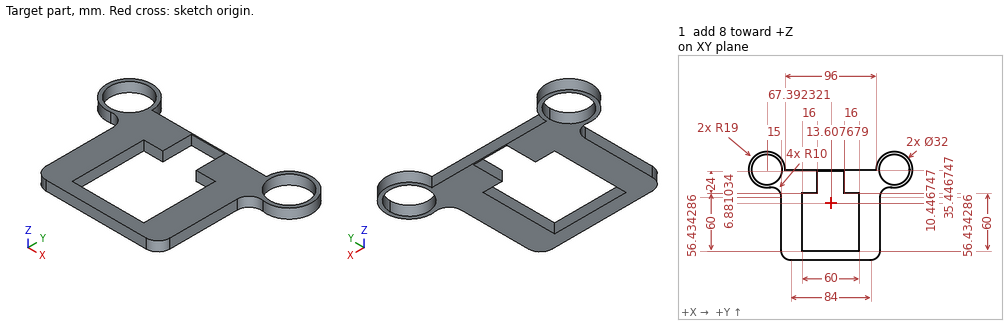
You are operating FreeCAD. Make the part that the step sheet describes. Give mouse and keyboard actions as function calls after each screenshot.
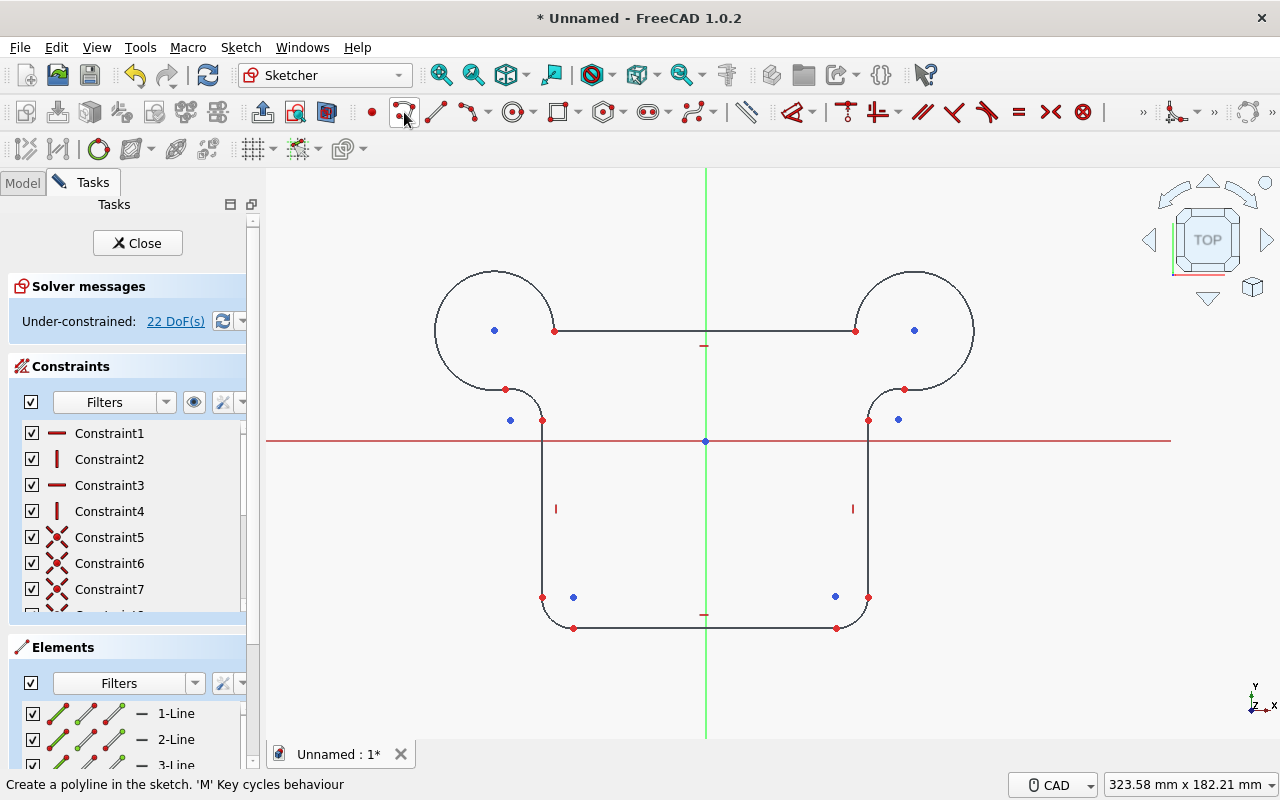
click(749, 409)
click(799, 409)
click(799, 597)
click(611, 597)
click(611, 409)
click(661, 409)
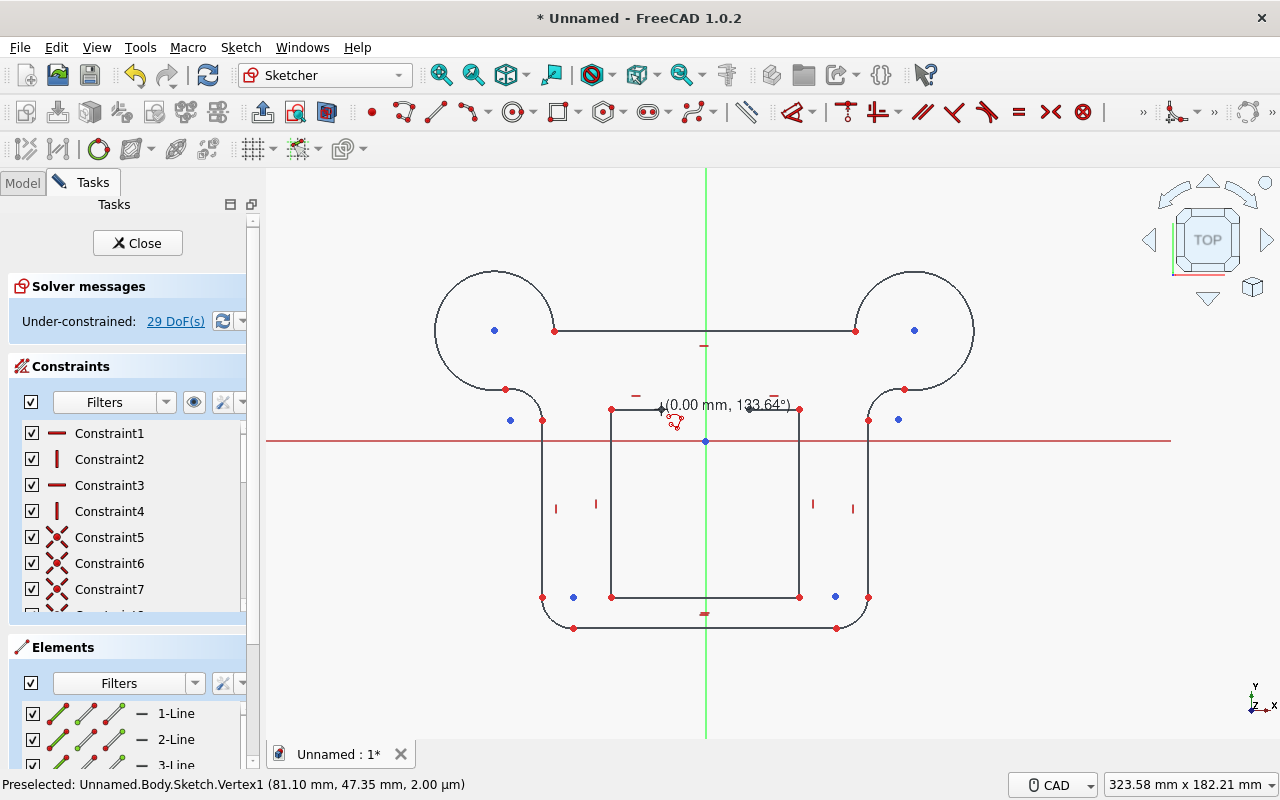
scroll(661, 333, up, 9)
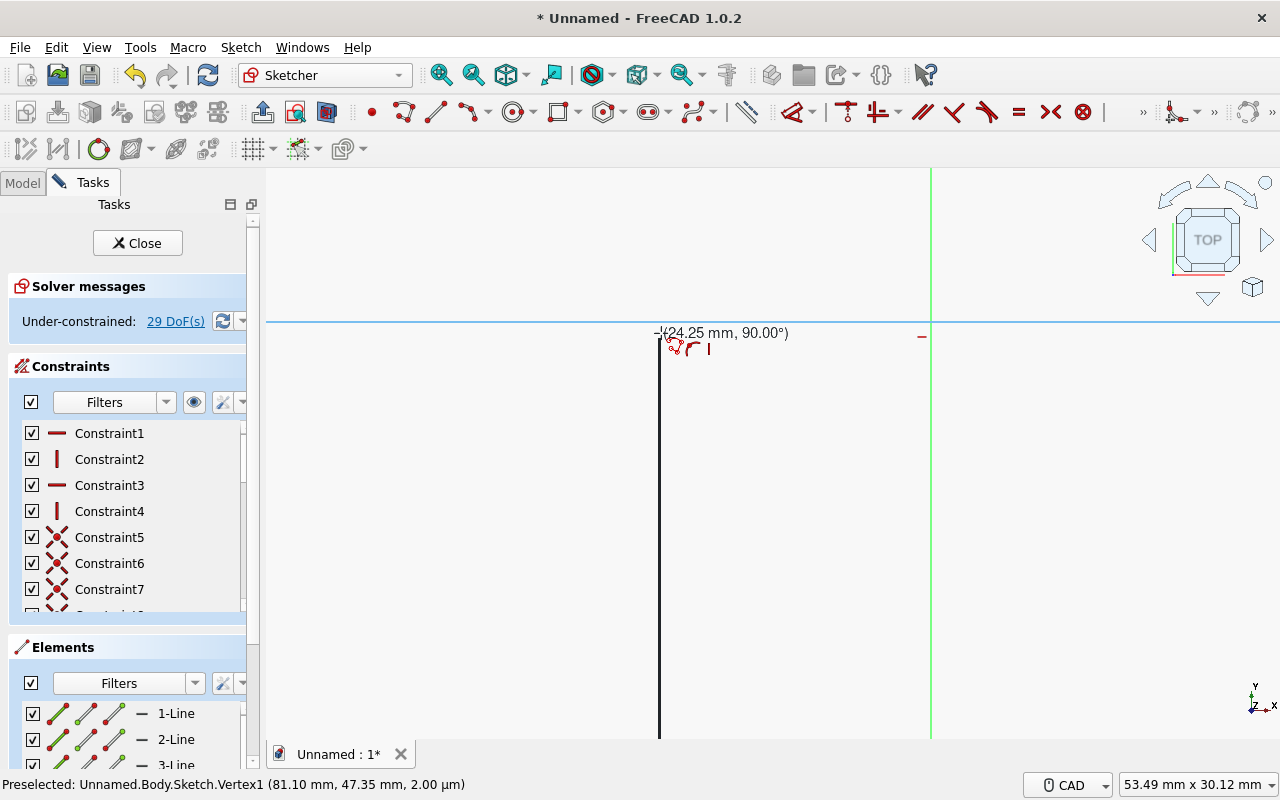
click(659, 334)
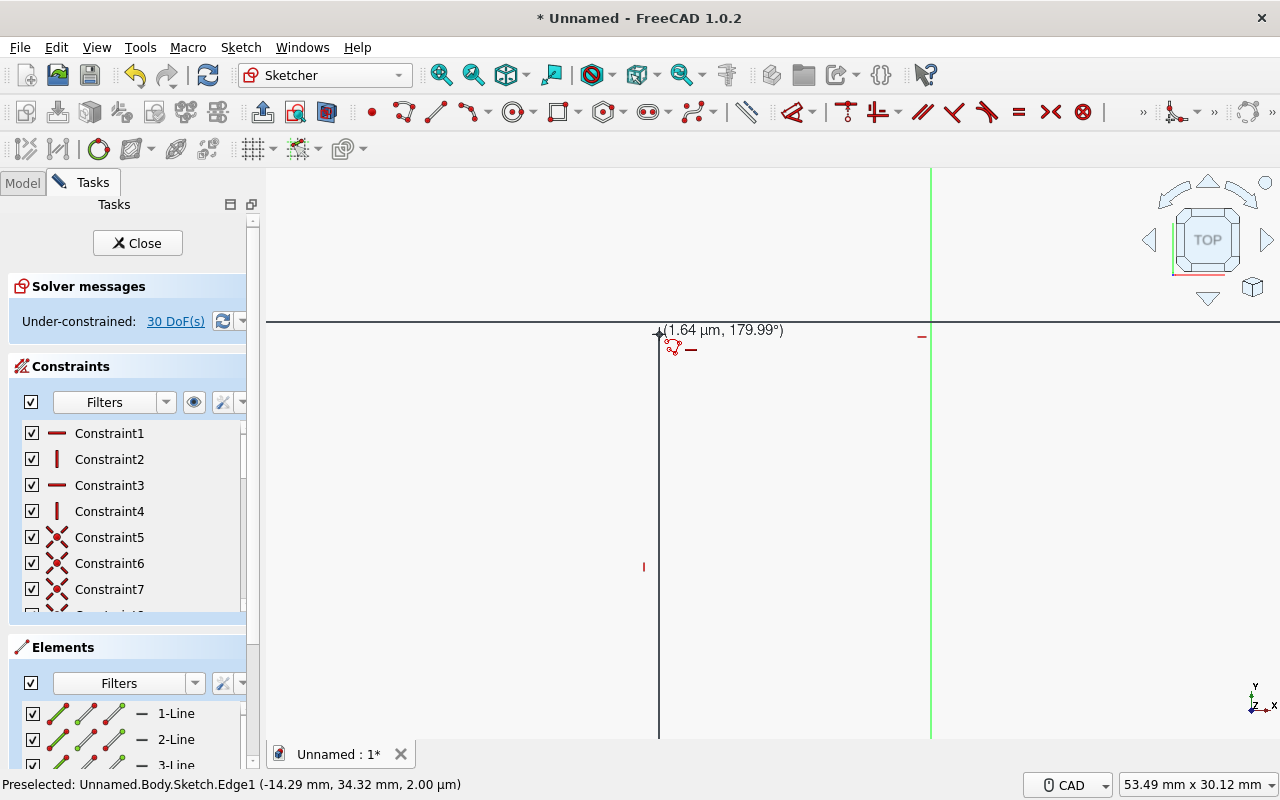
scroll(661, 333, down, 9)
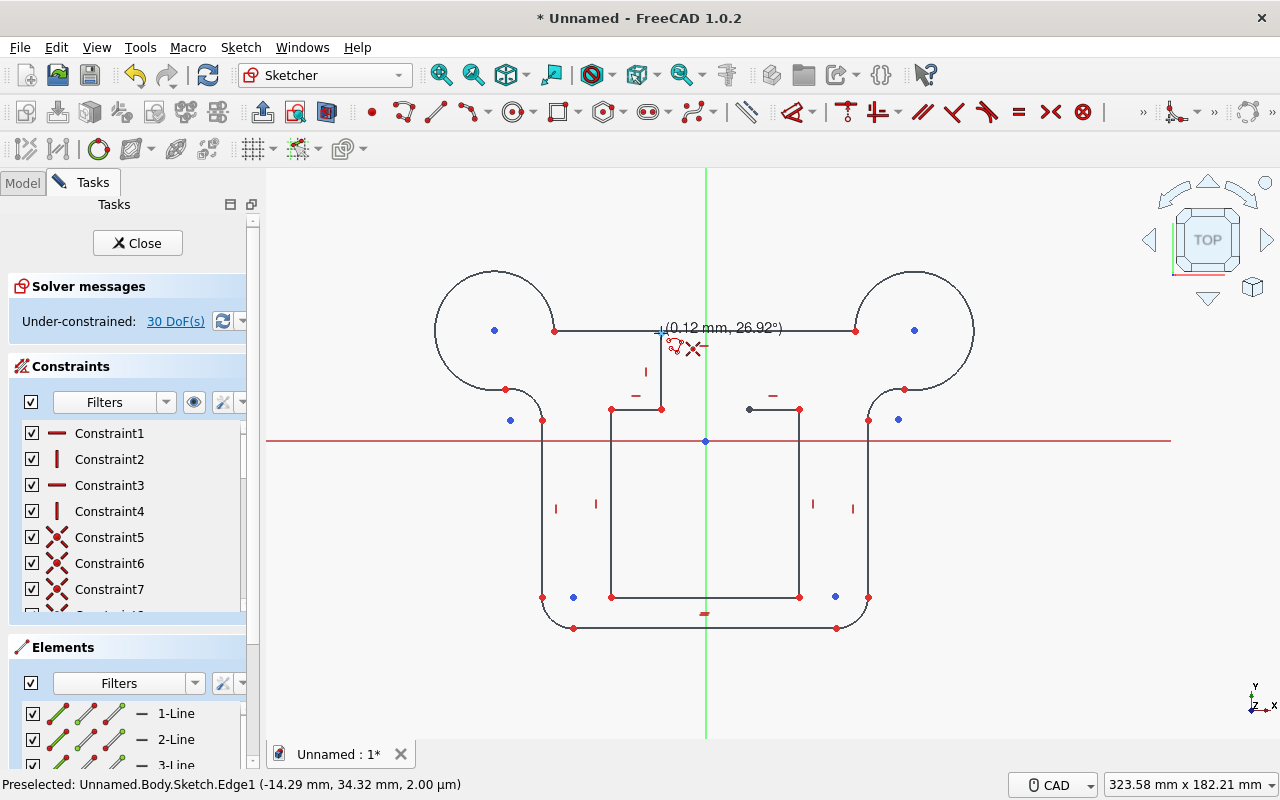
scroll(749, 333, up, 9)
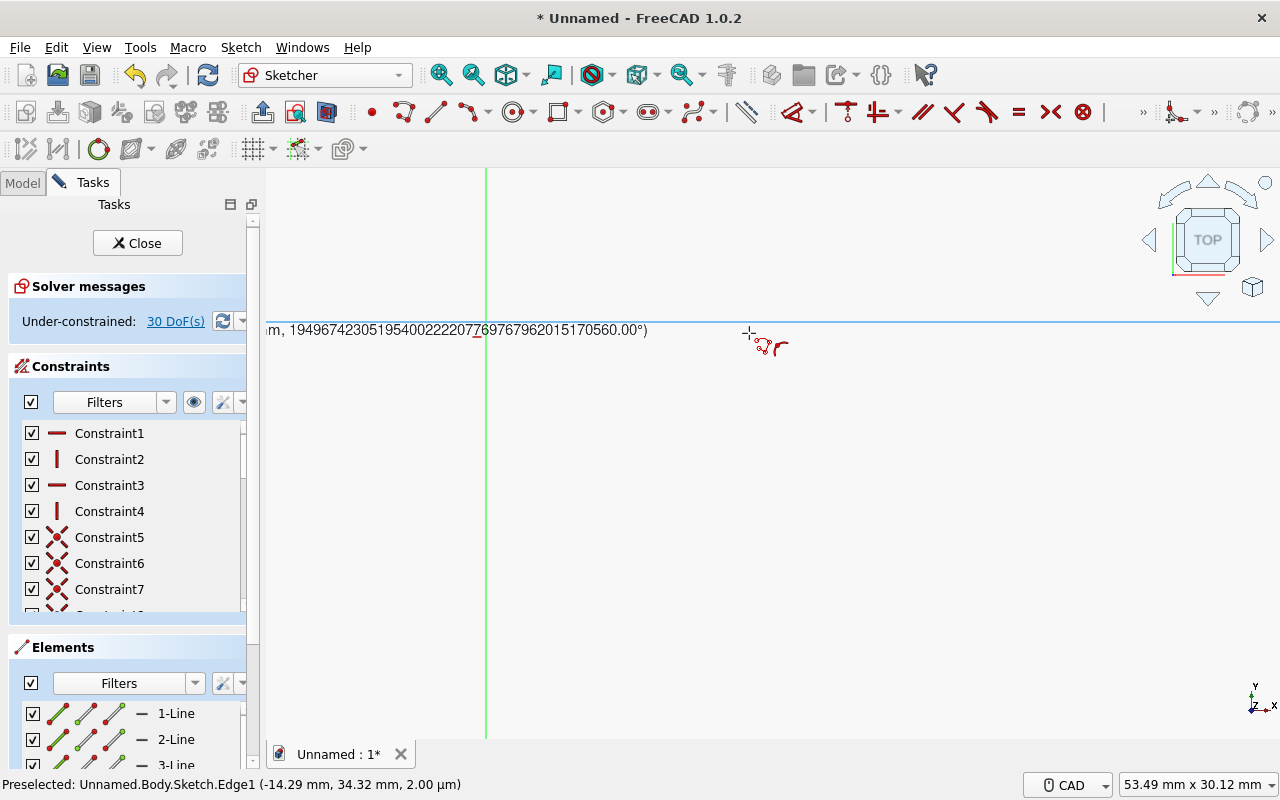
click(744, 334)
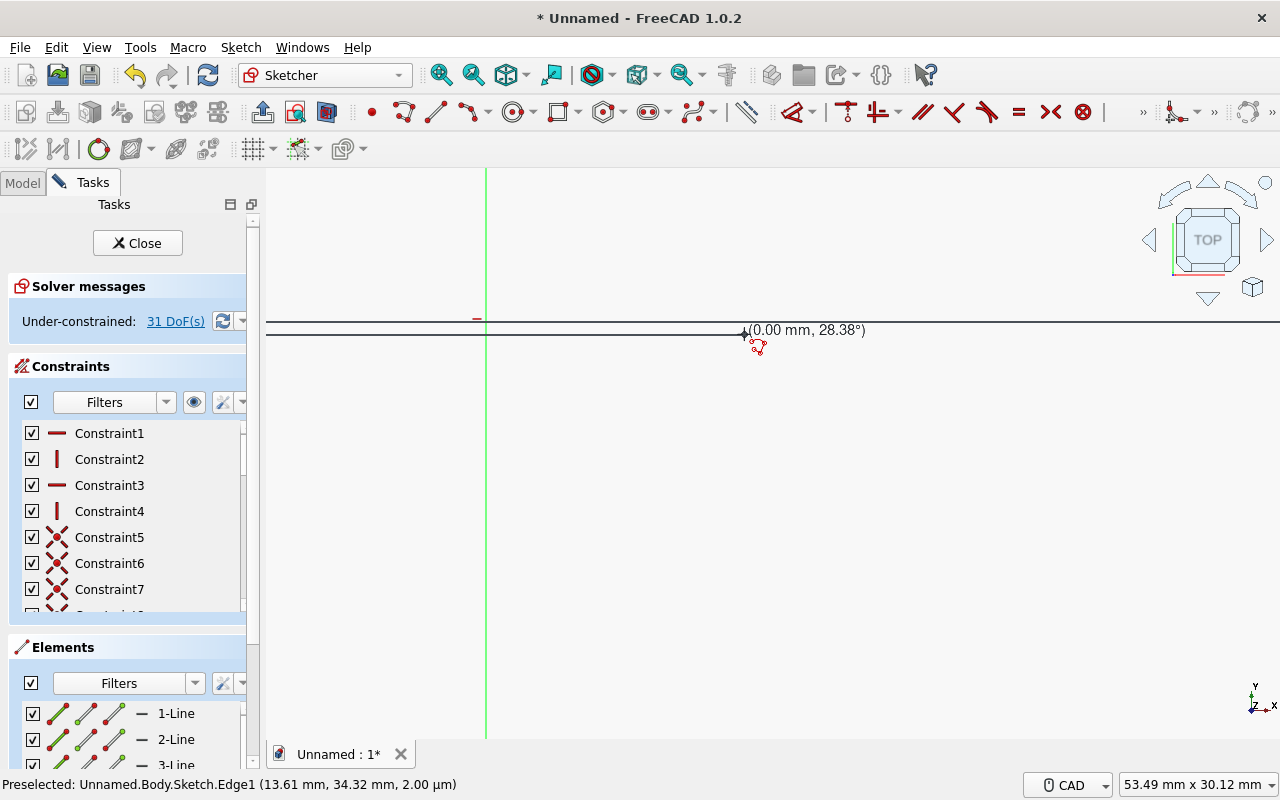
scroll(749, 333, down, 9)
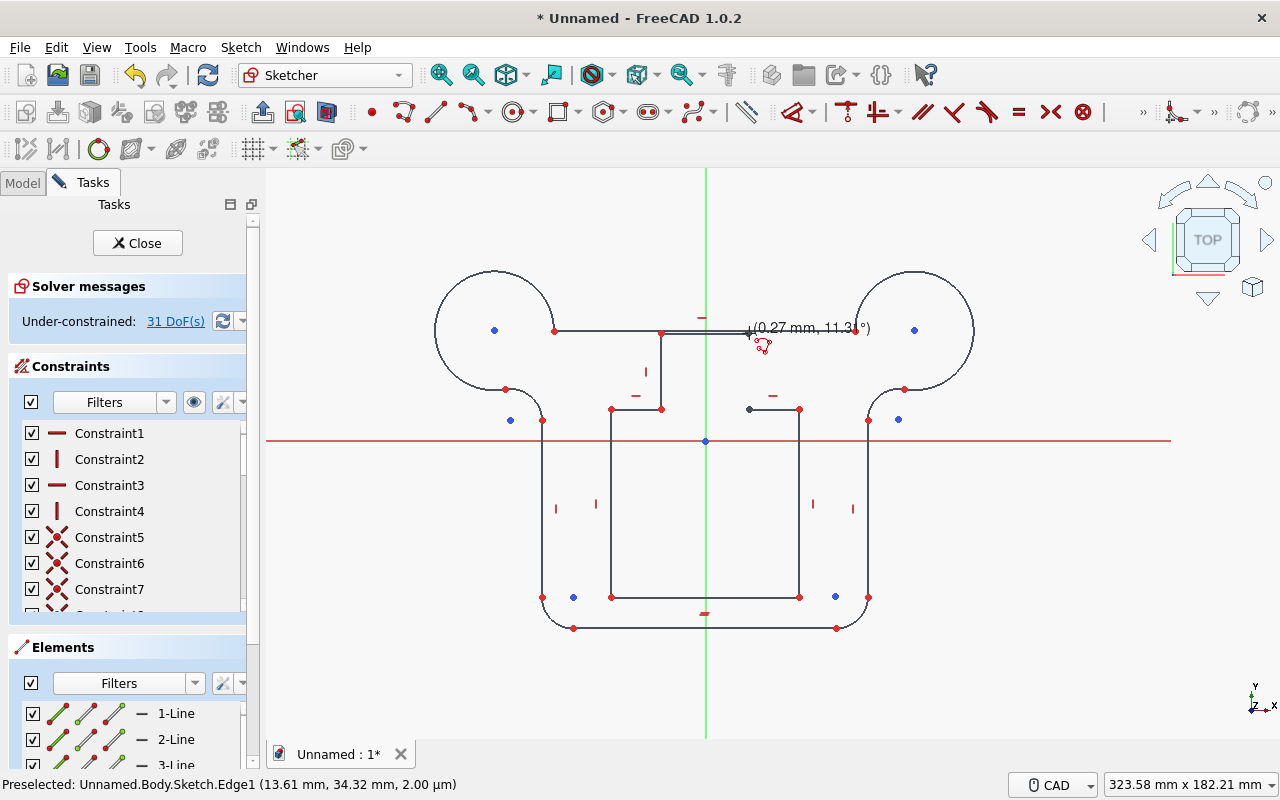
click(749, 410)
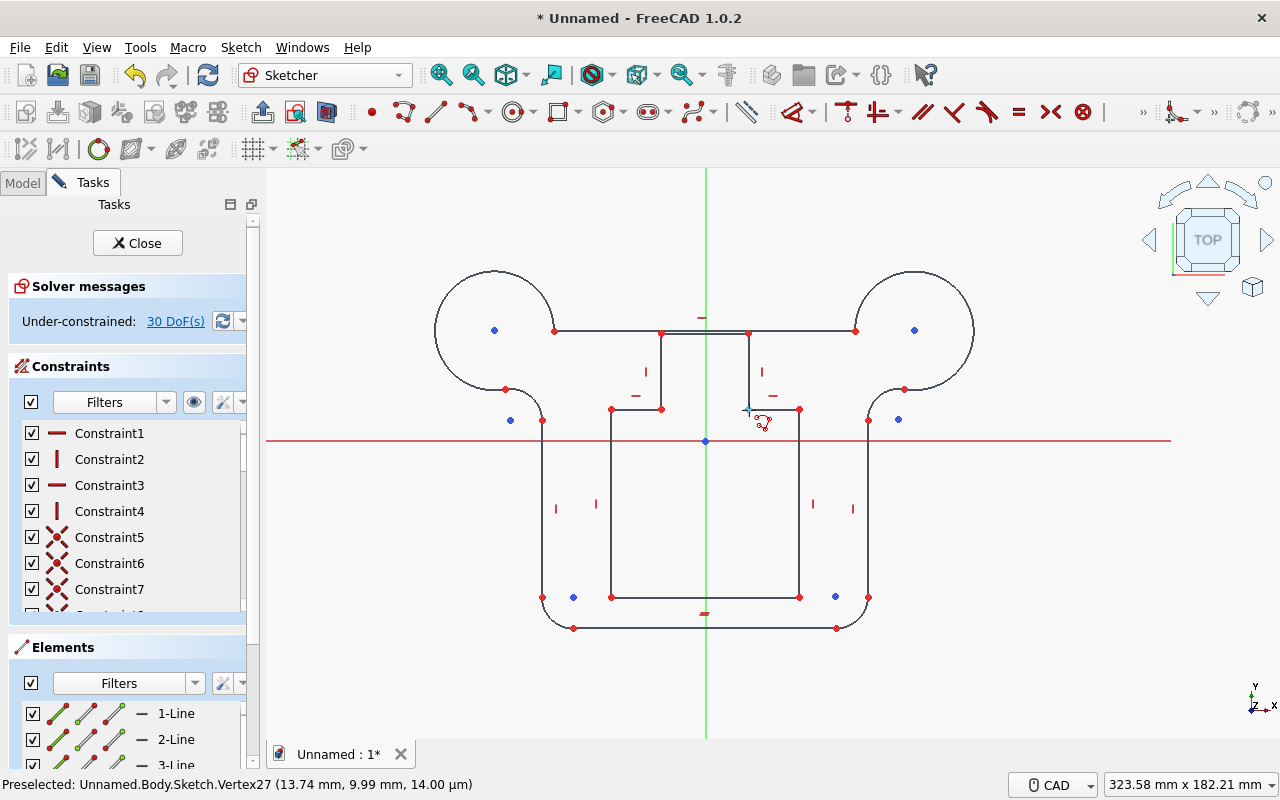
click(514, 112)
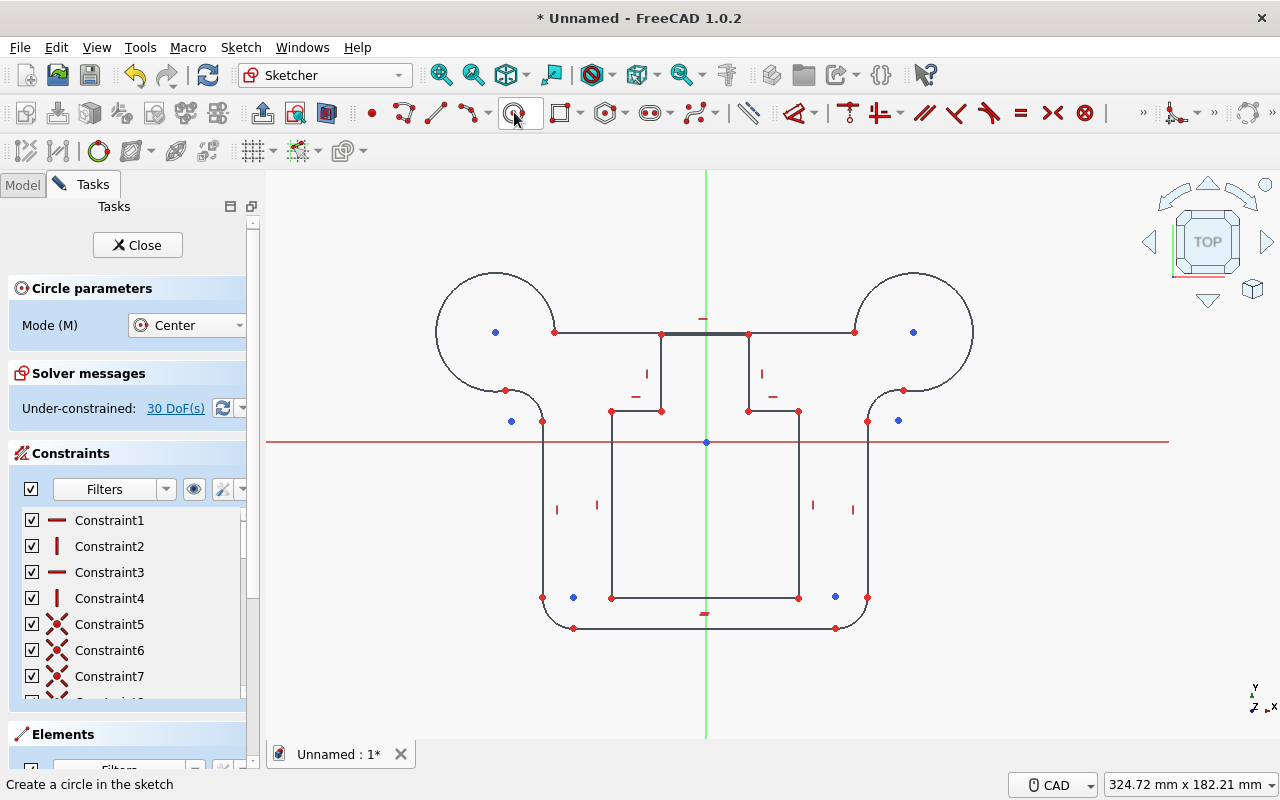
click(496, 332)
move(531, 367)